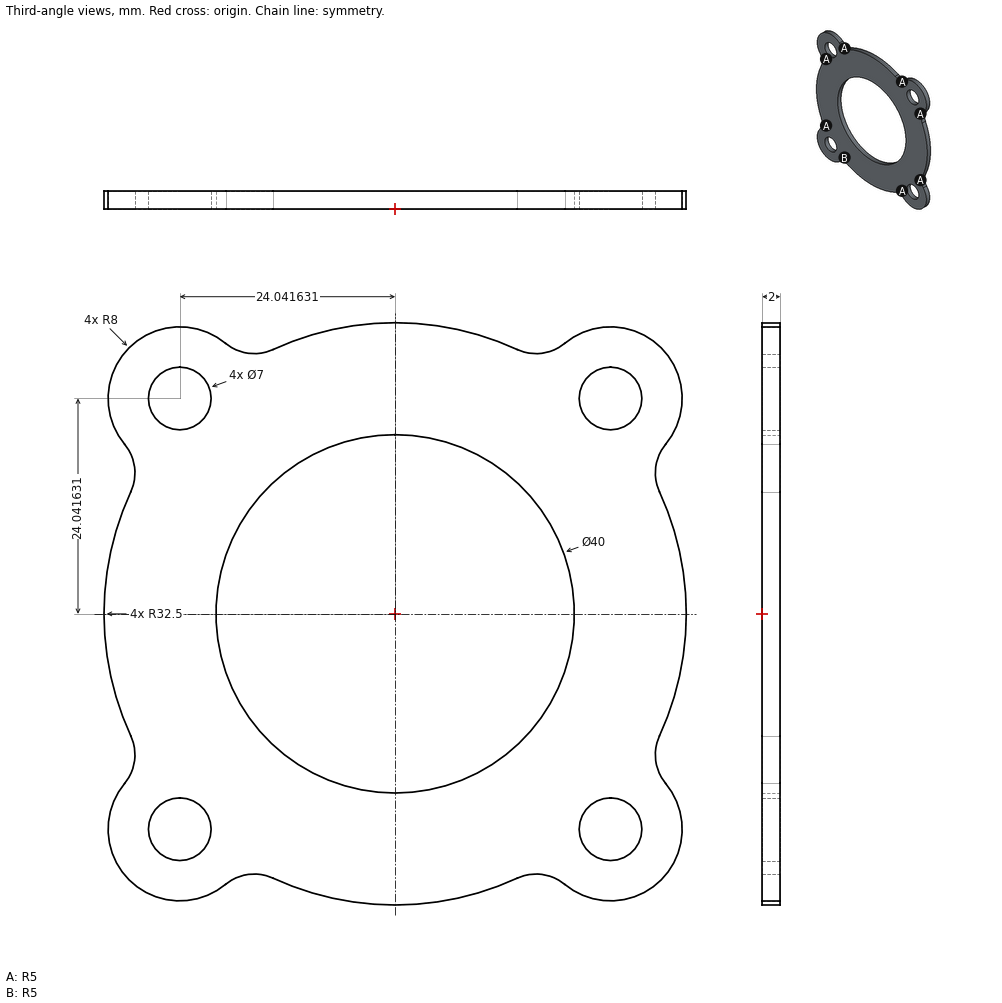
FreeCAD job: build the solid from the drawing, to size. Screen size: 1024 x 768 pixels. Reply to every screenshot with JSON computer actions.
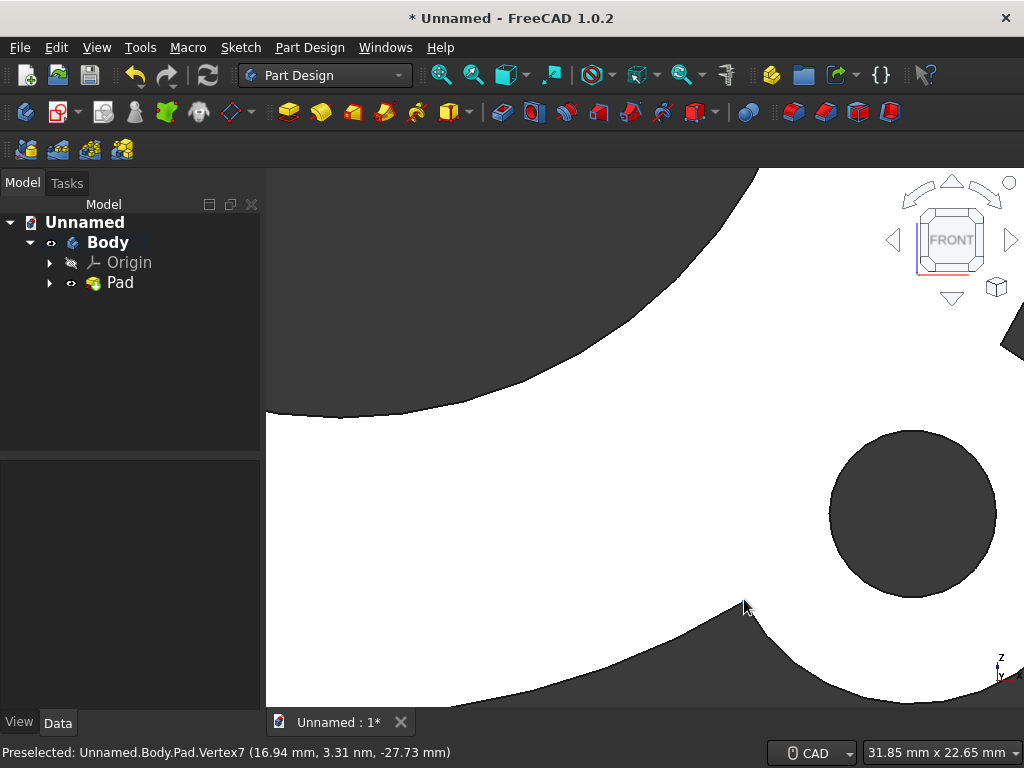
{"action": "left_click", "coordinate": [442, 76]}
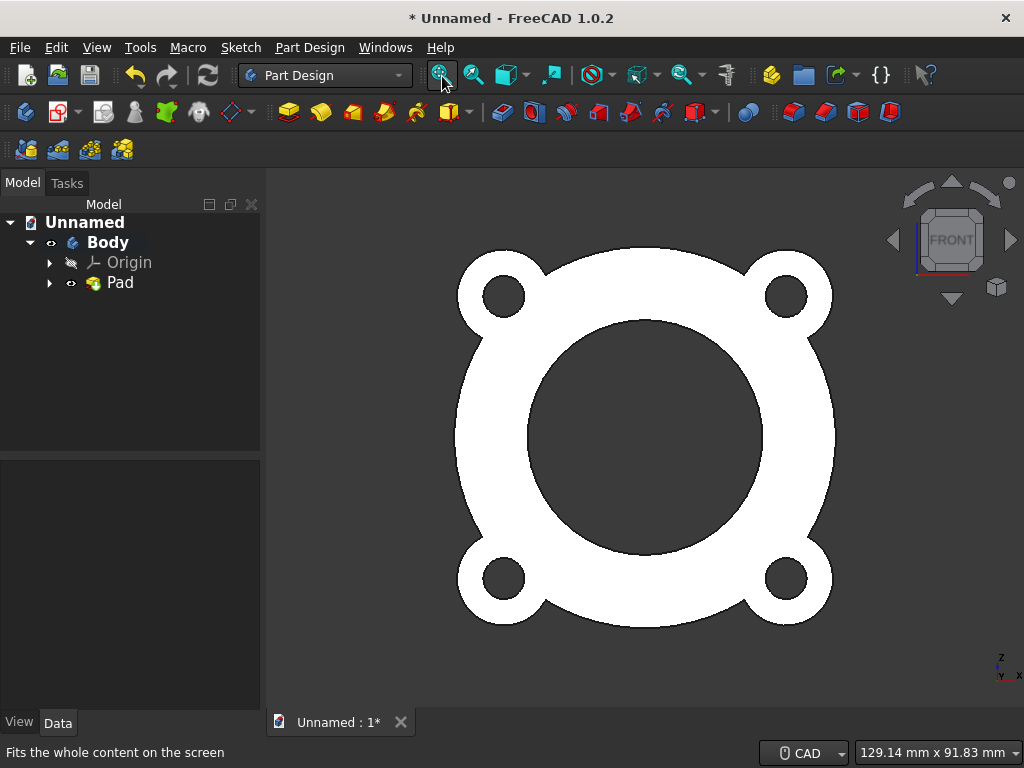
{"action": "key", "text": "3"}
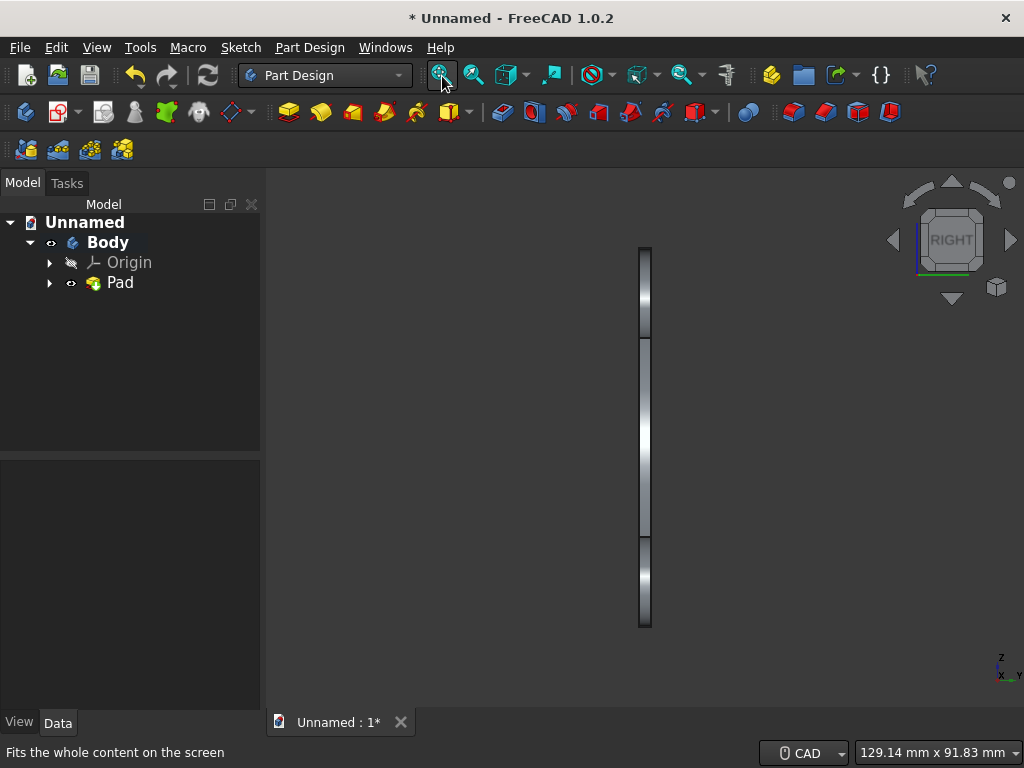
{"action": "scroll", "coordinate": [645, 599], "scroll_direction": "up", "scroll_amount": 7}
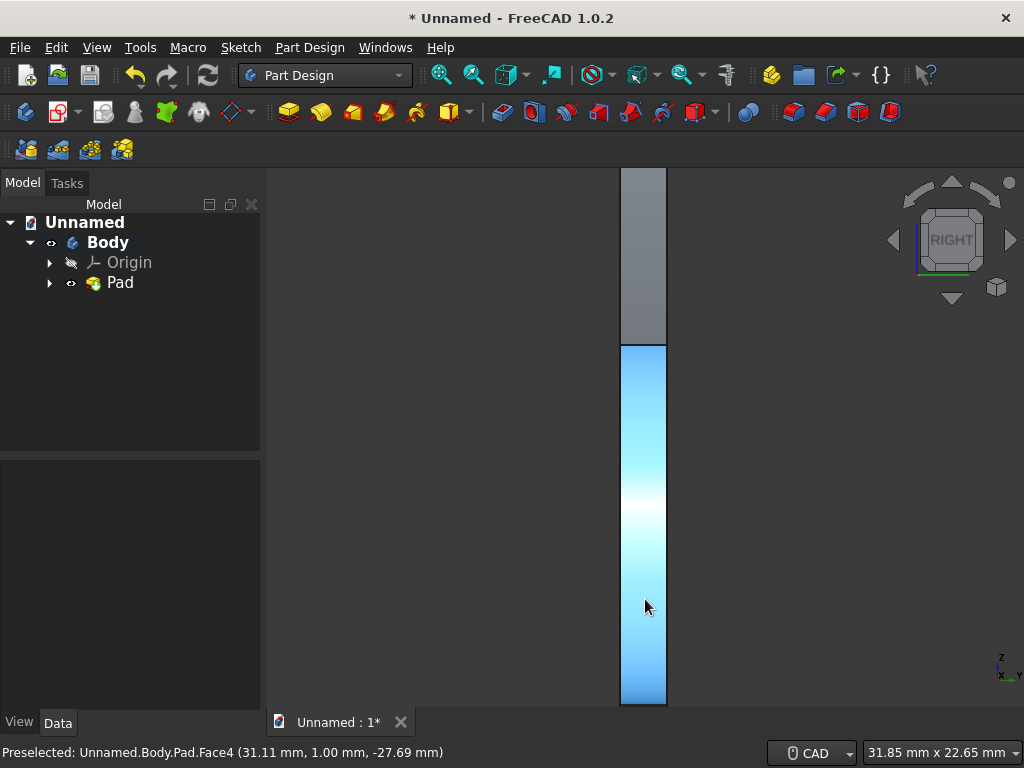
{"action": "left_click", "coordinate": [442, 76]}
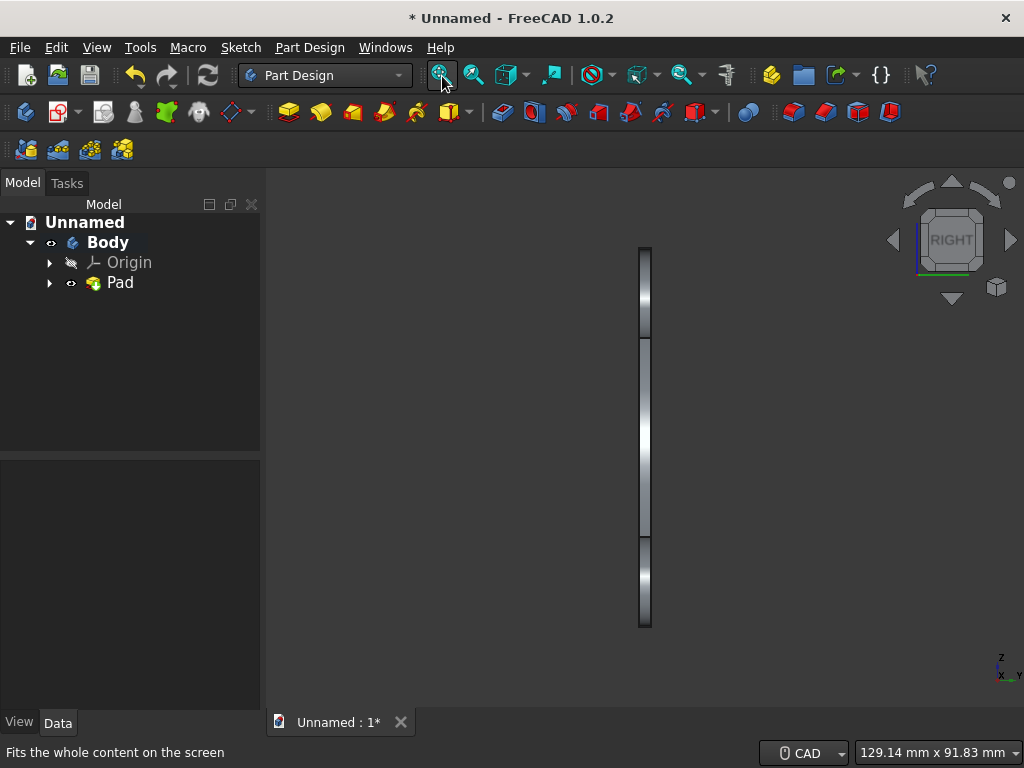
{"action": "key", "text": "5"}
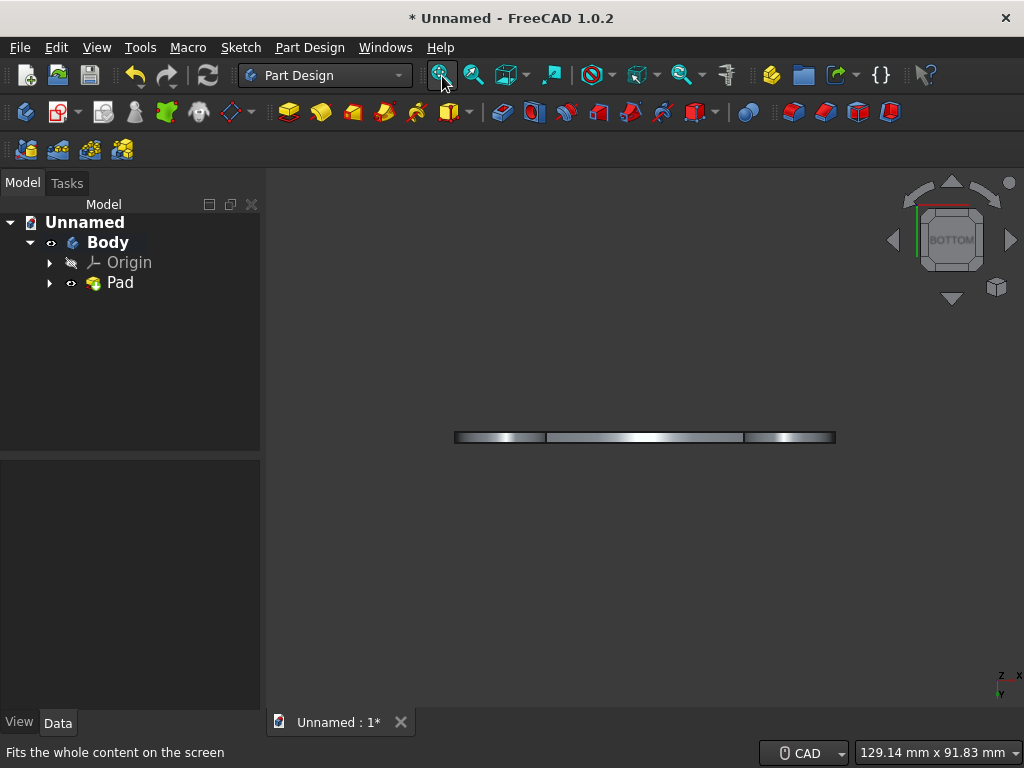
{"action": "scroll", "coordinate": [744, 436], "scroll_direction": "up", "scroll_amount": 7}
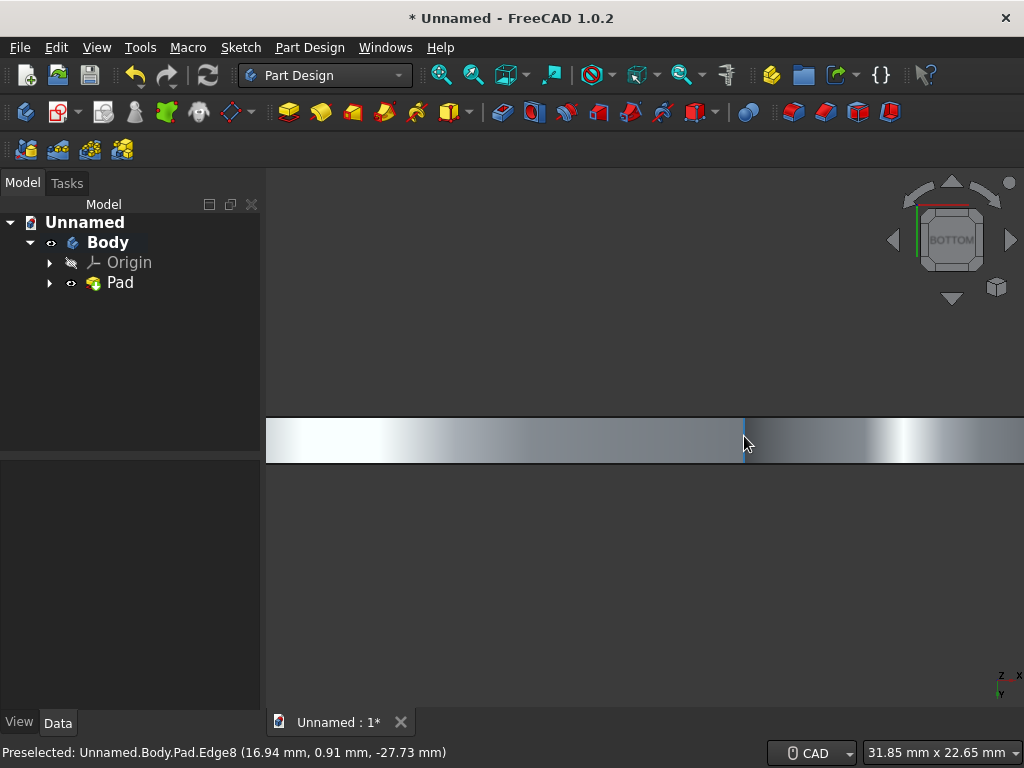
{"action": "left_click", "coordinate": [442, 76]}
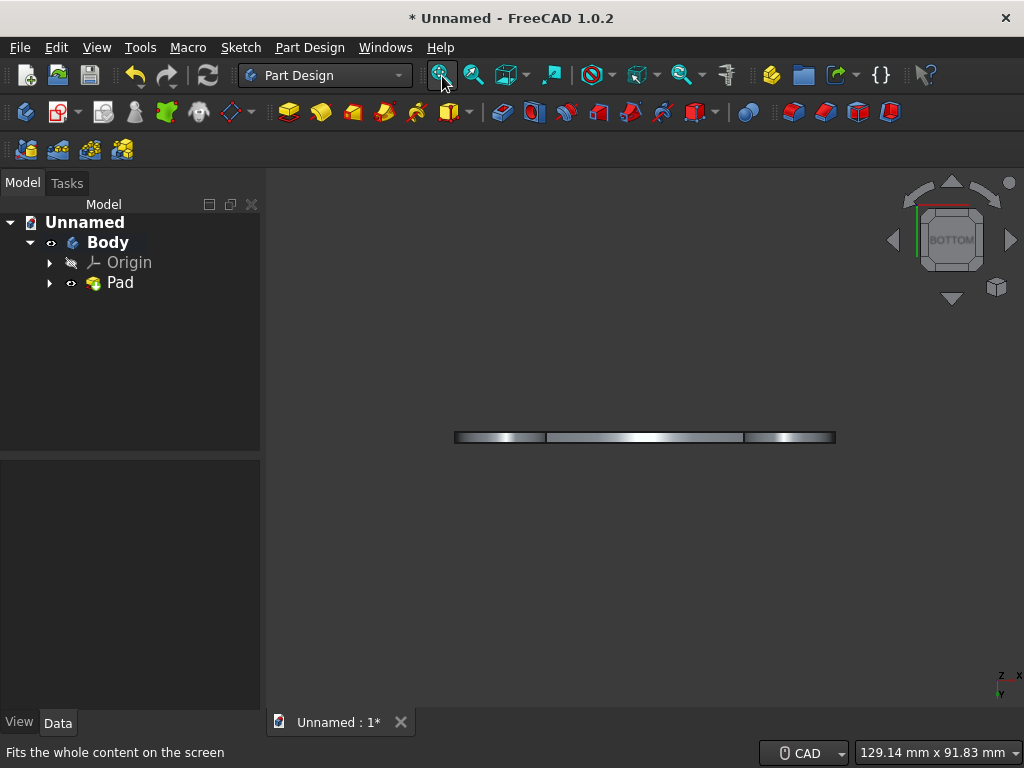
{"action": "key", "text": "4"}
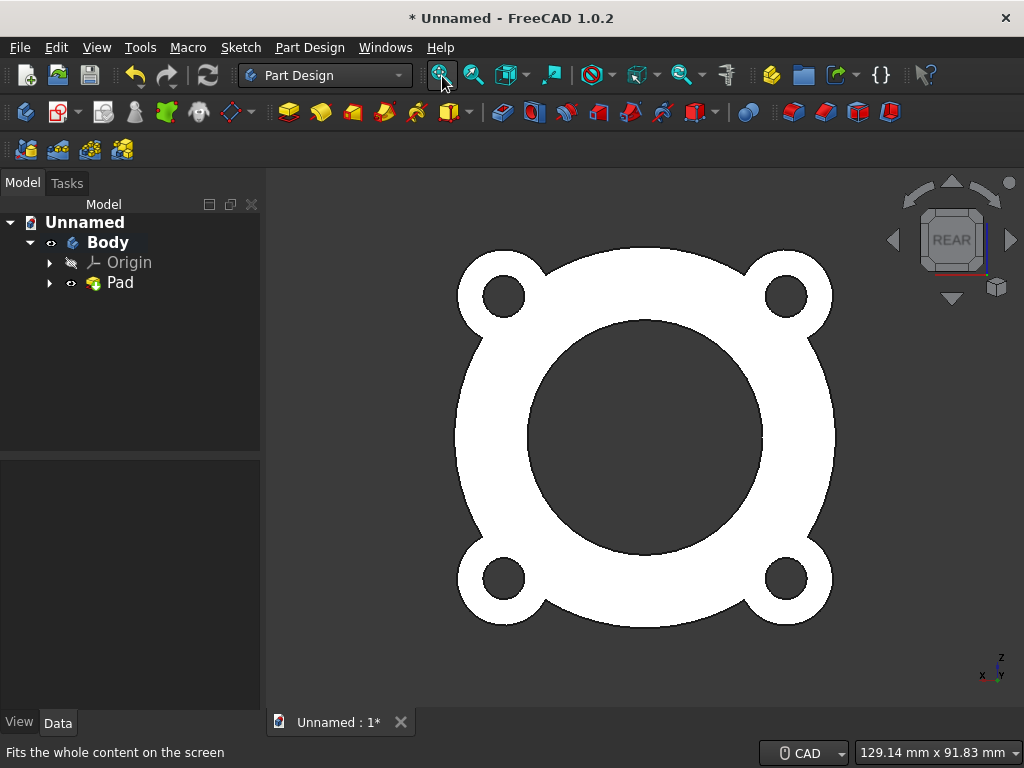
{"action": "scroll", "coordinate": [546, 599], "scroll_direction": "up", "scroll_amount": 7}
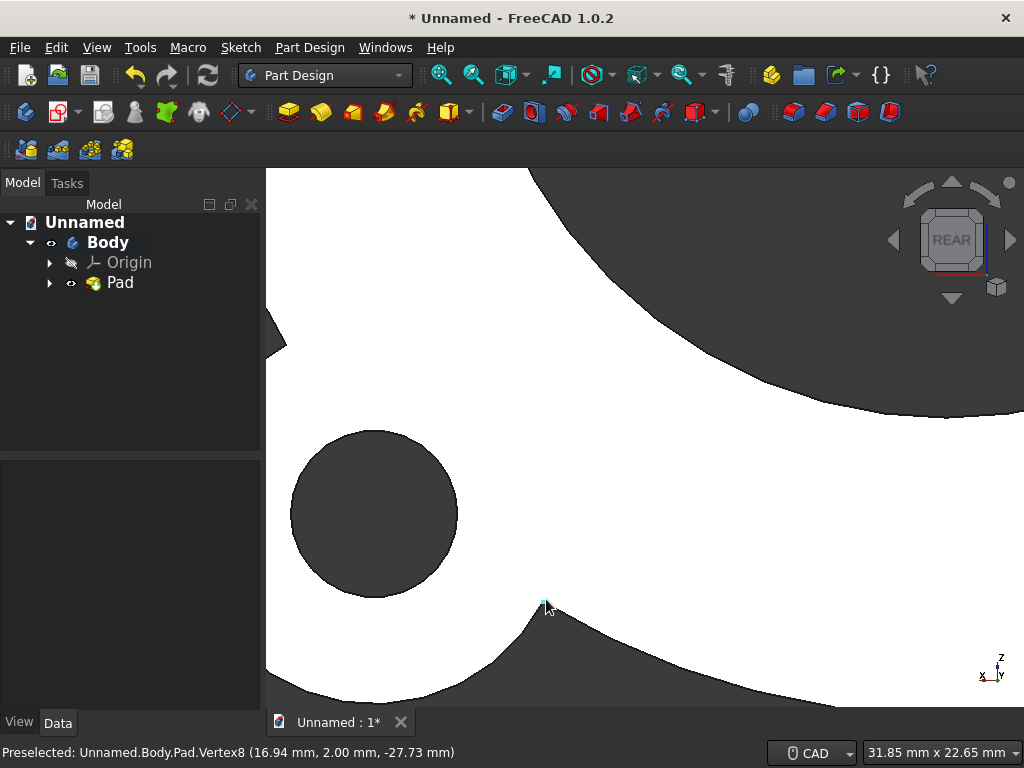
{"action": "key", "text": "v f"}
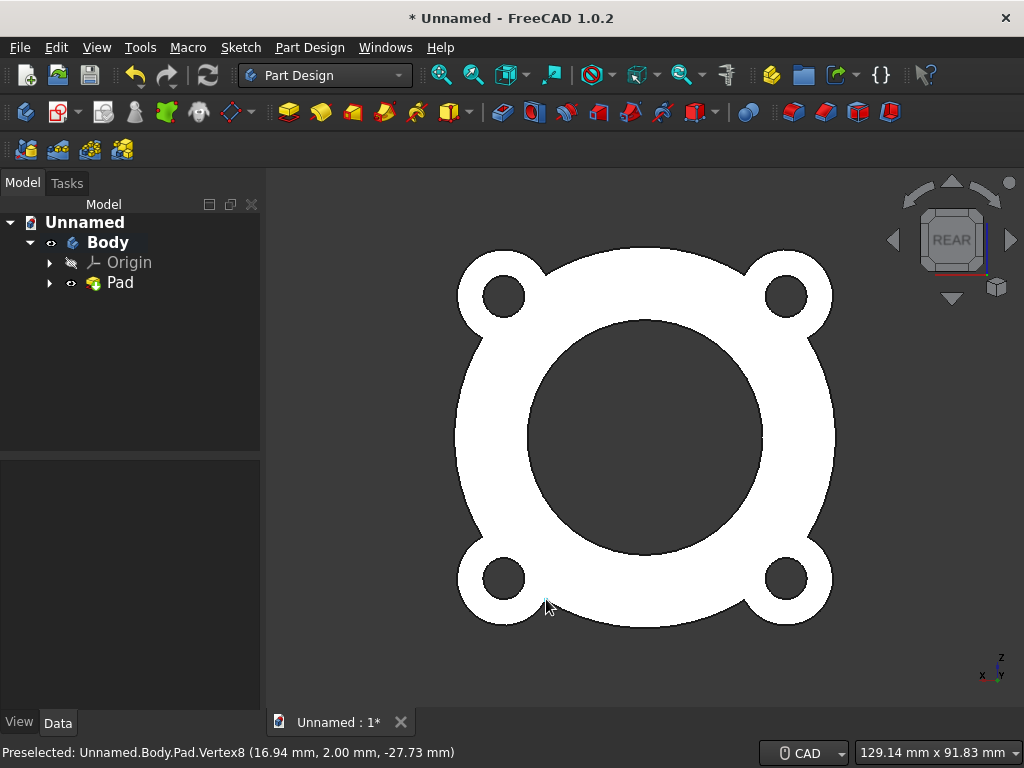
{"action": "key", "text": "6"}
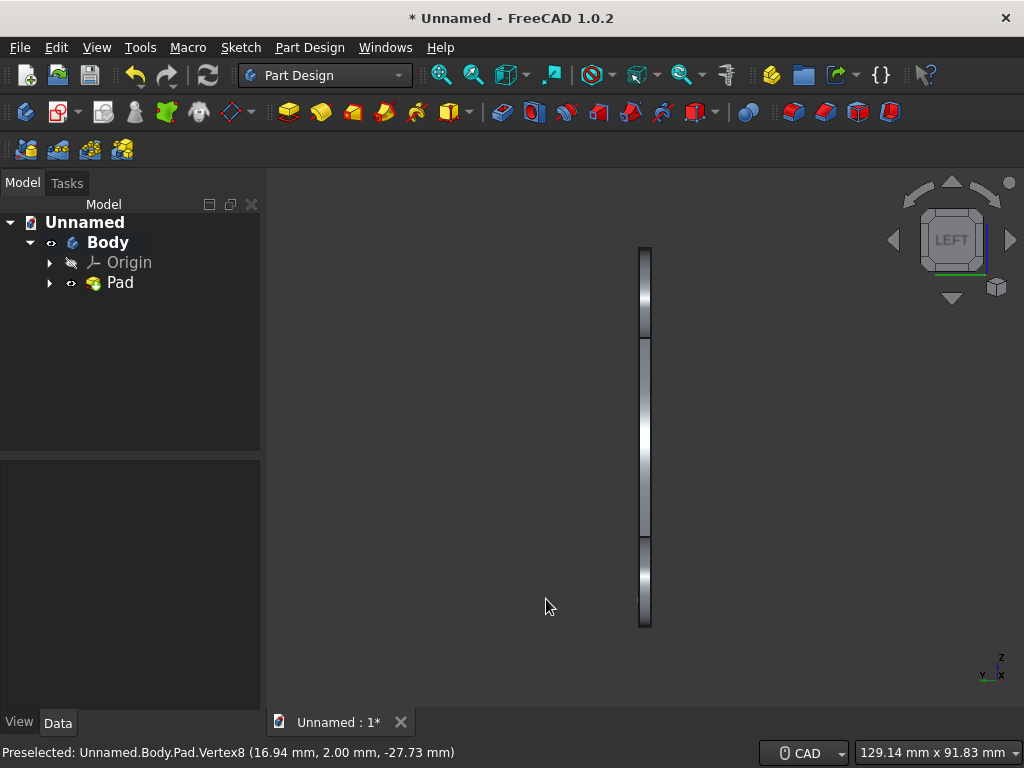
{"action": "scroll", "coordinate": [645, 599], "scroll_direction": "up", "scroll_amount": 7}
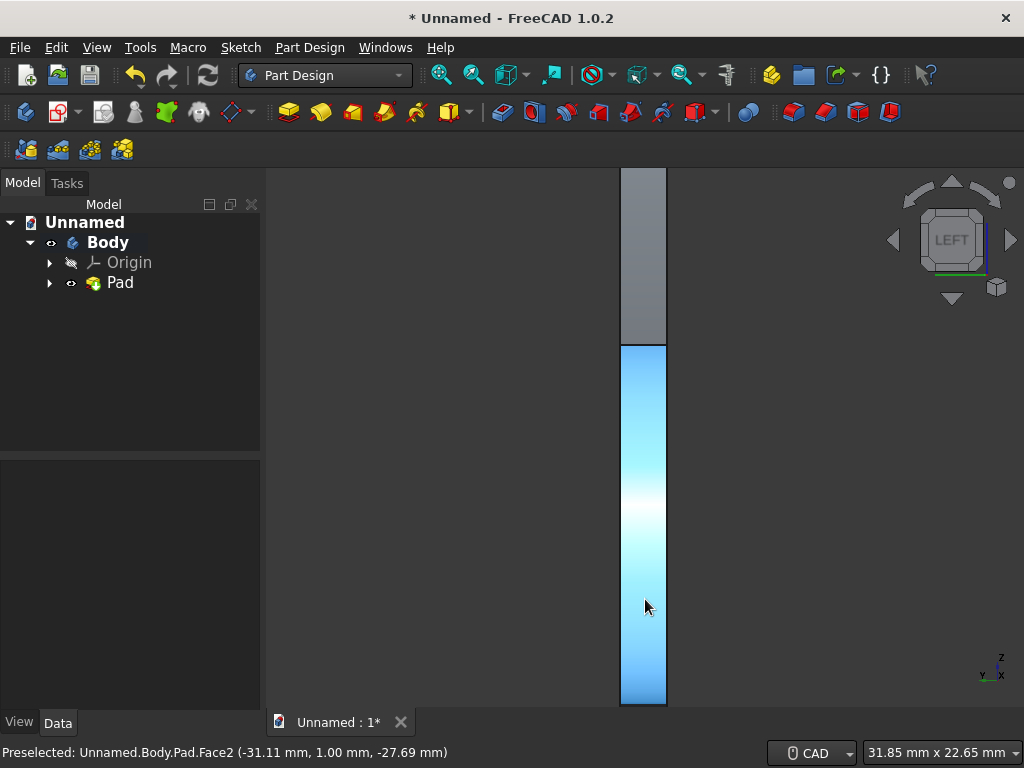
{"action": "left_click", "coordinate": [442, 76]}